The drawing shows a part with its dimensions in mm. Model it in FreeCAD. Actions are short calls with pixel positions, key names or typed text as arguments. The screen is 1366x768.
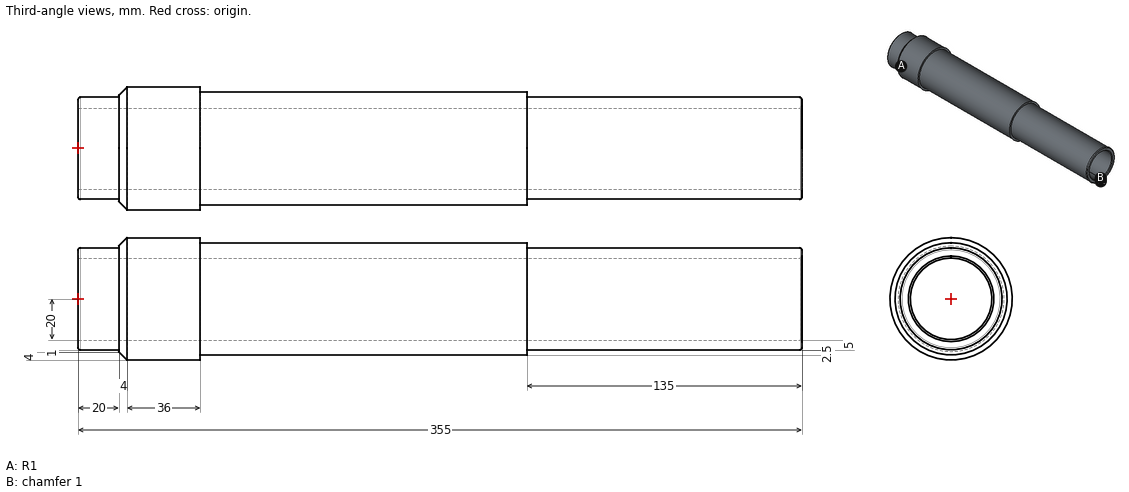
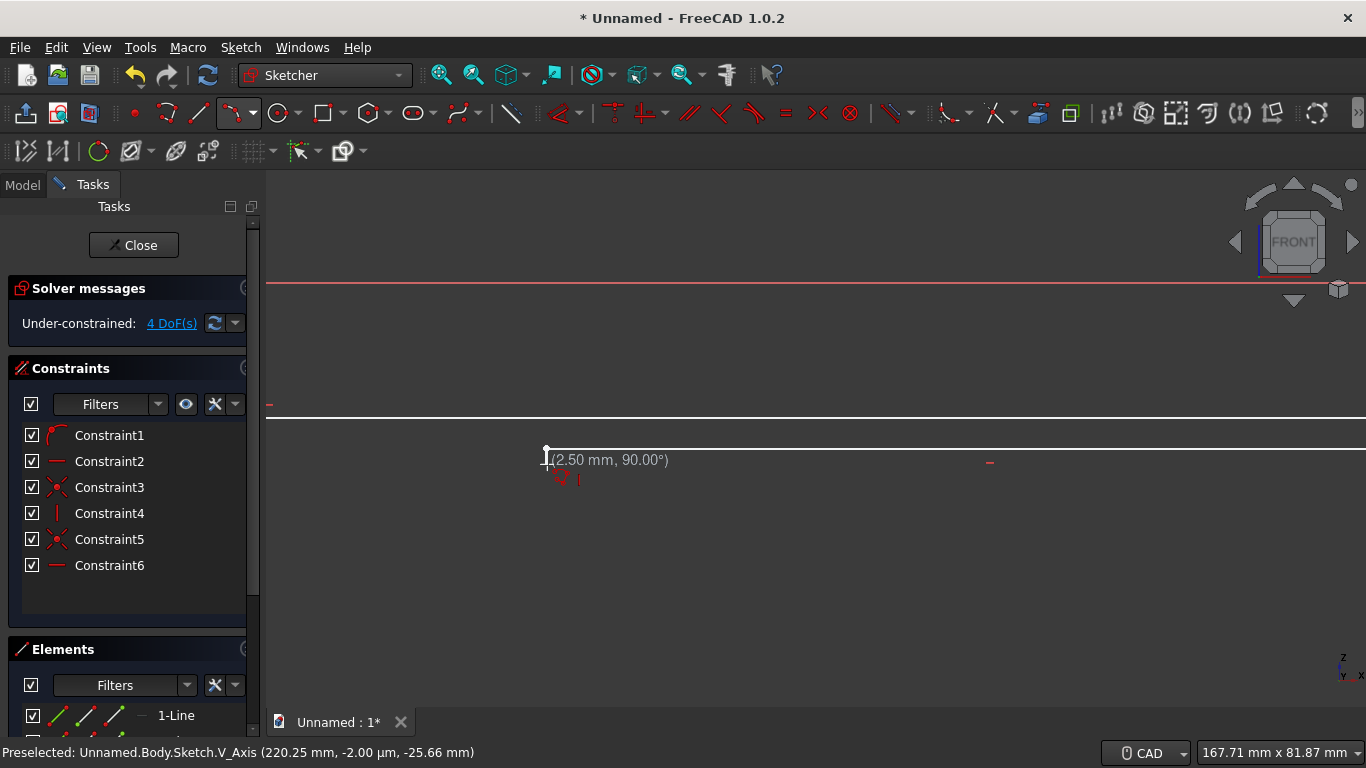
click(547, 463)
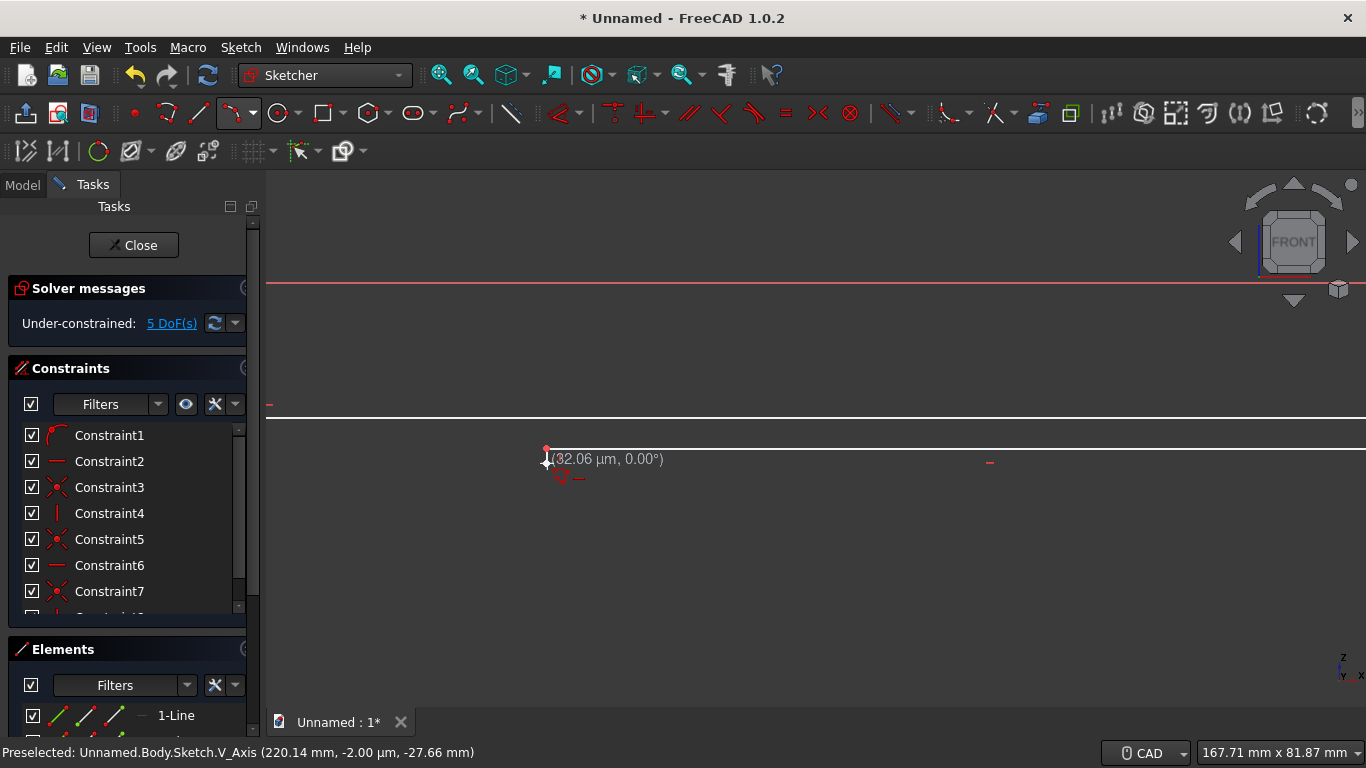
scroll(954, 463, down, 6)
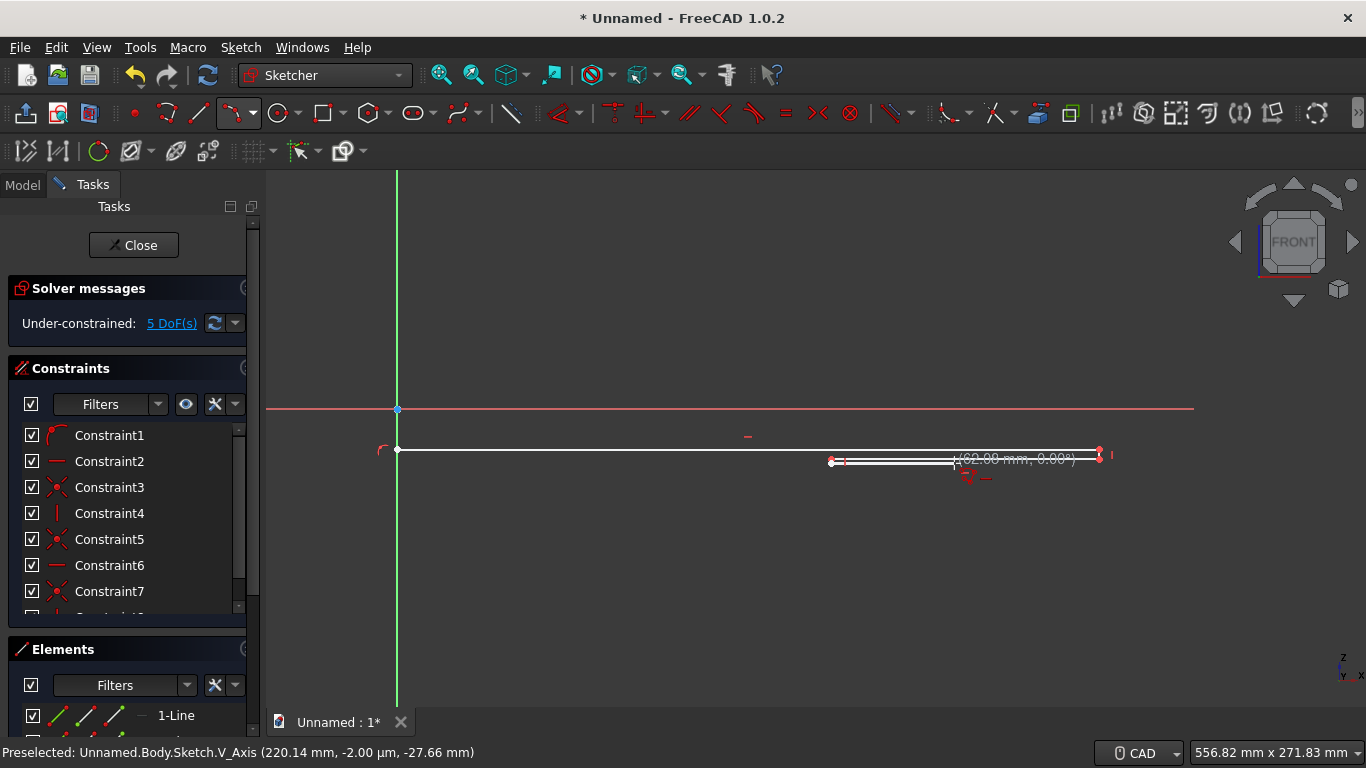
click(516, 463)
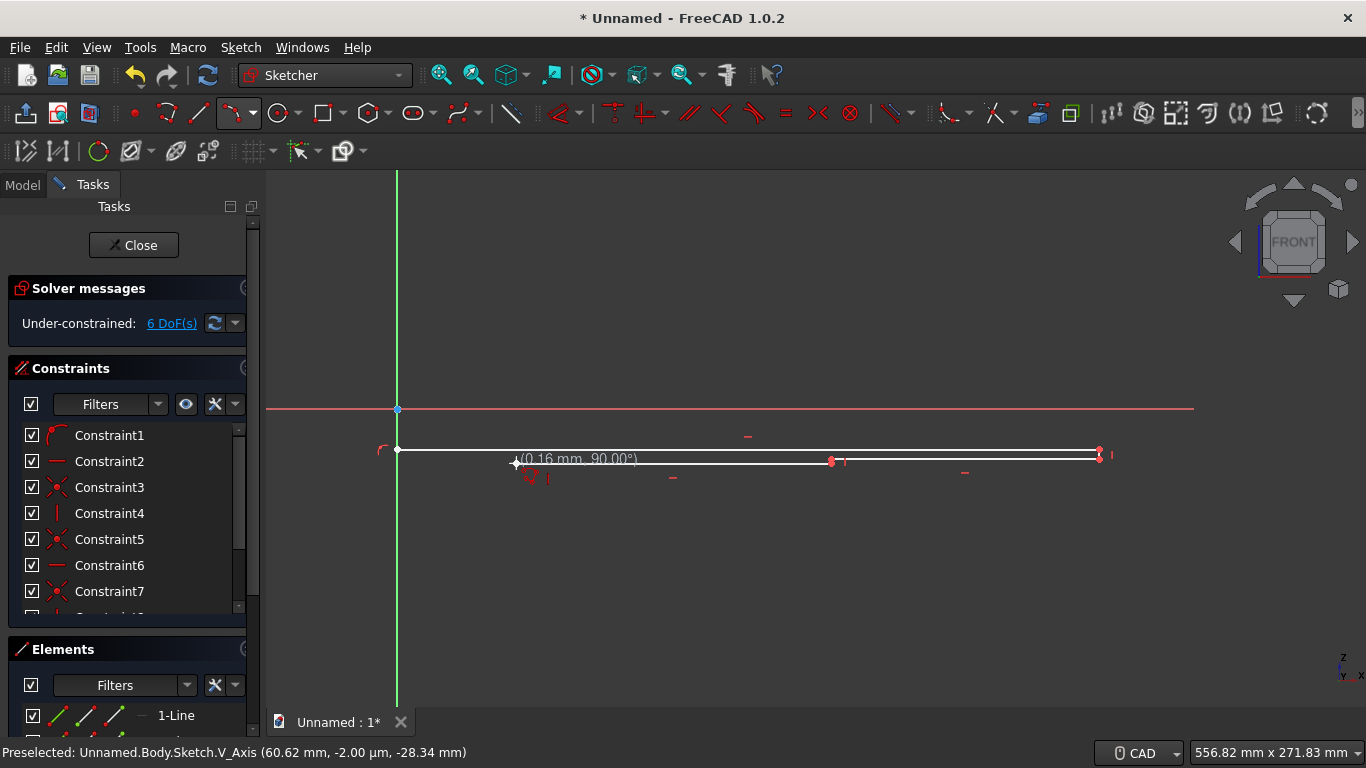
scroll(516, 468, up, 6)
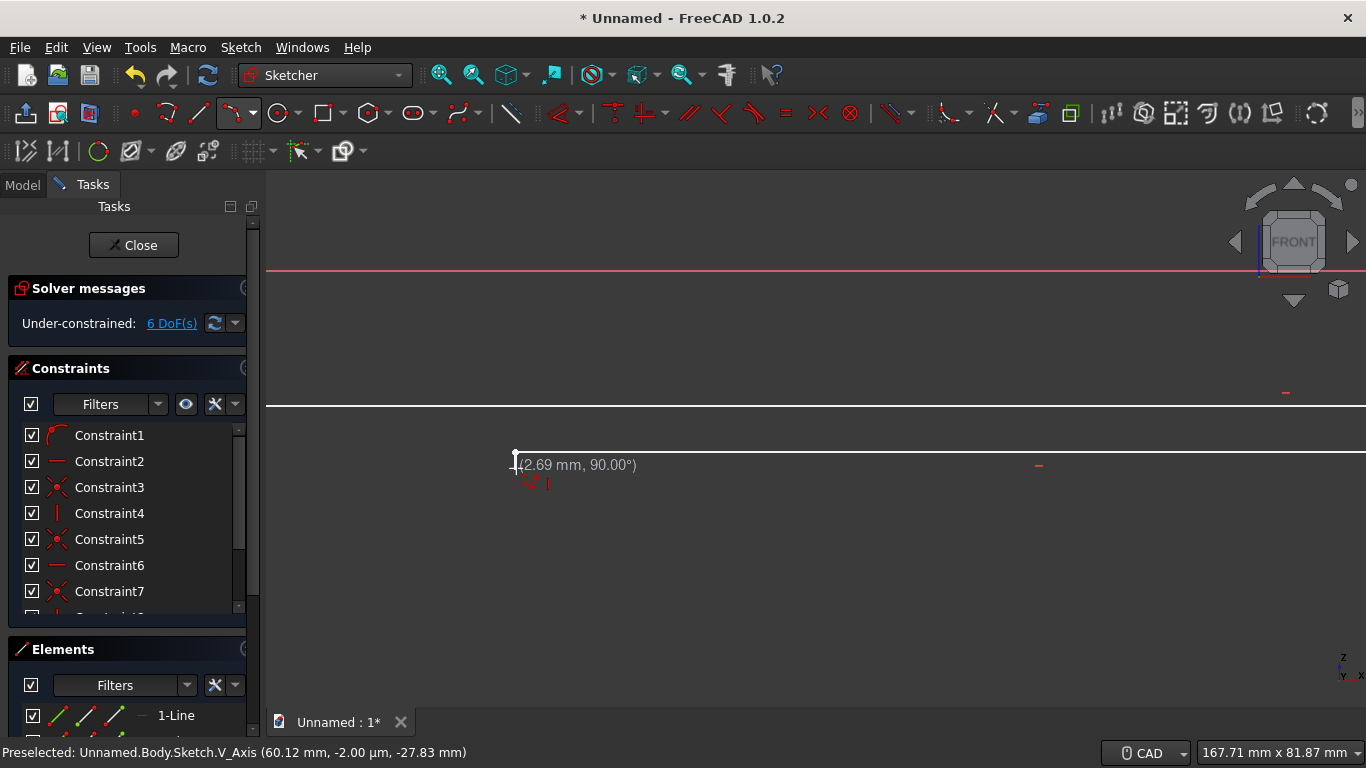
click(515, 468)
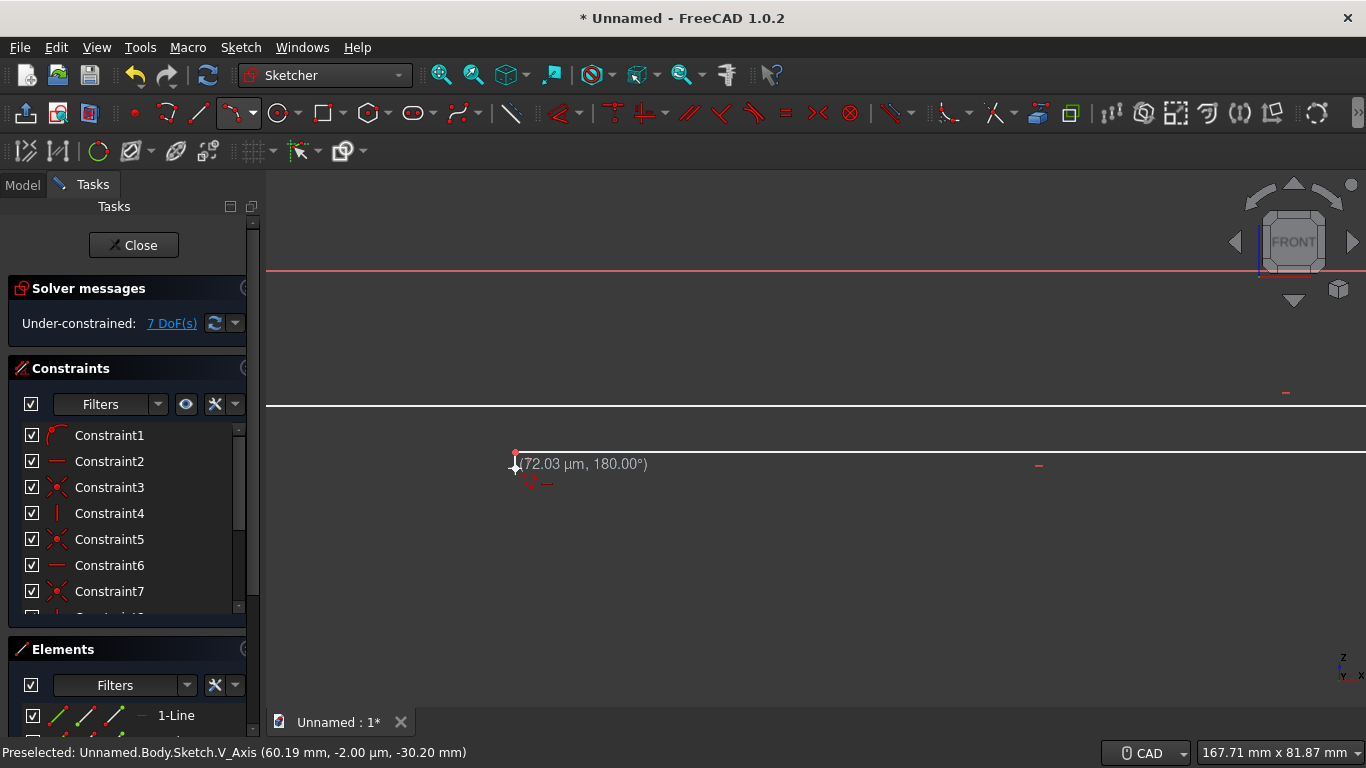
scroll(516, 468, down, 6)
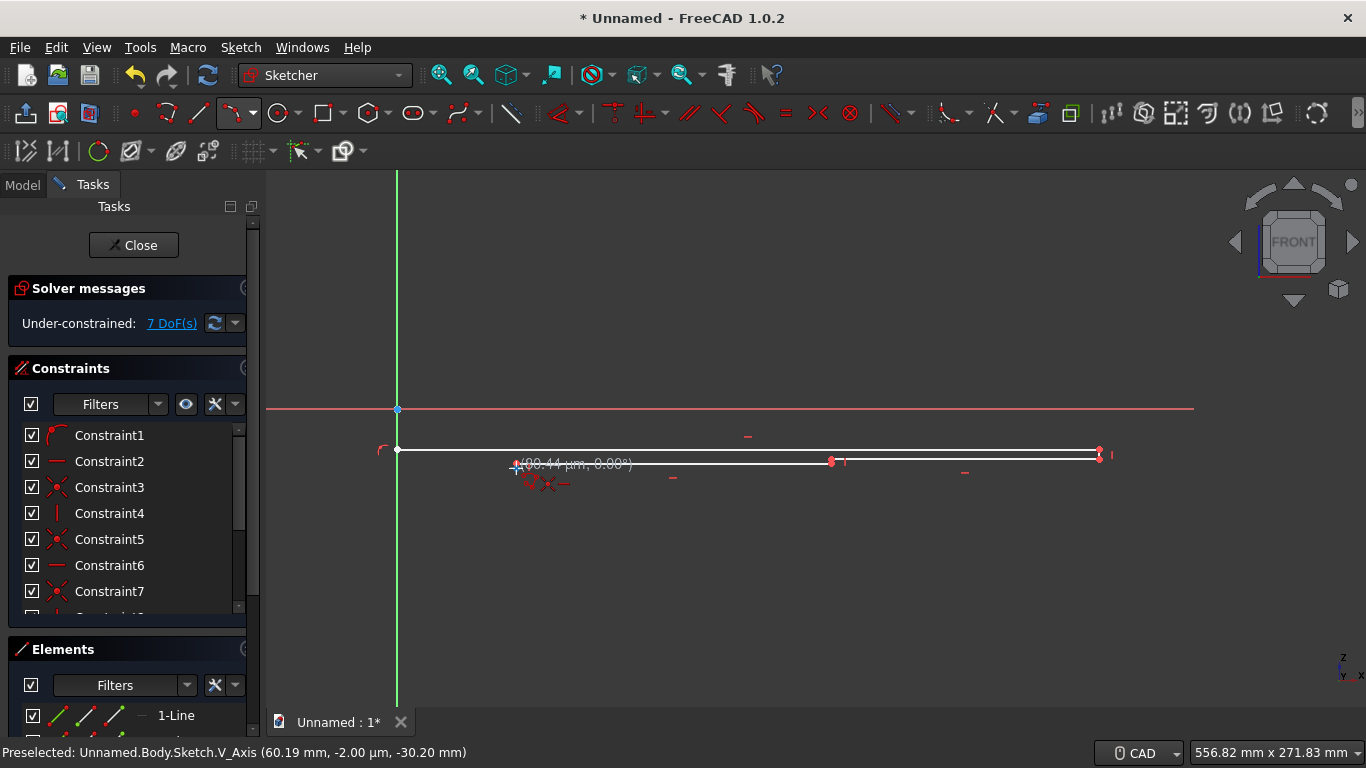
click(445, 468)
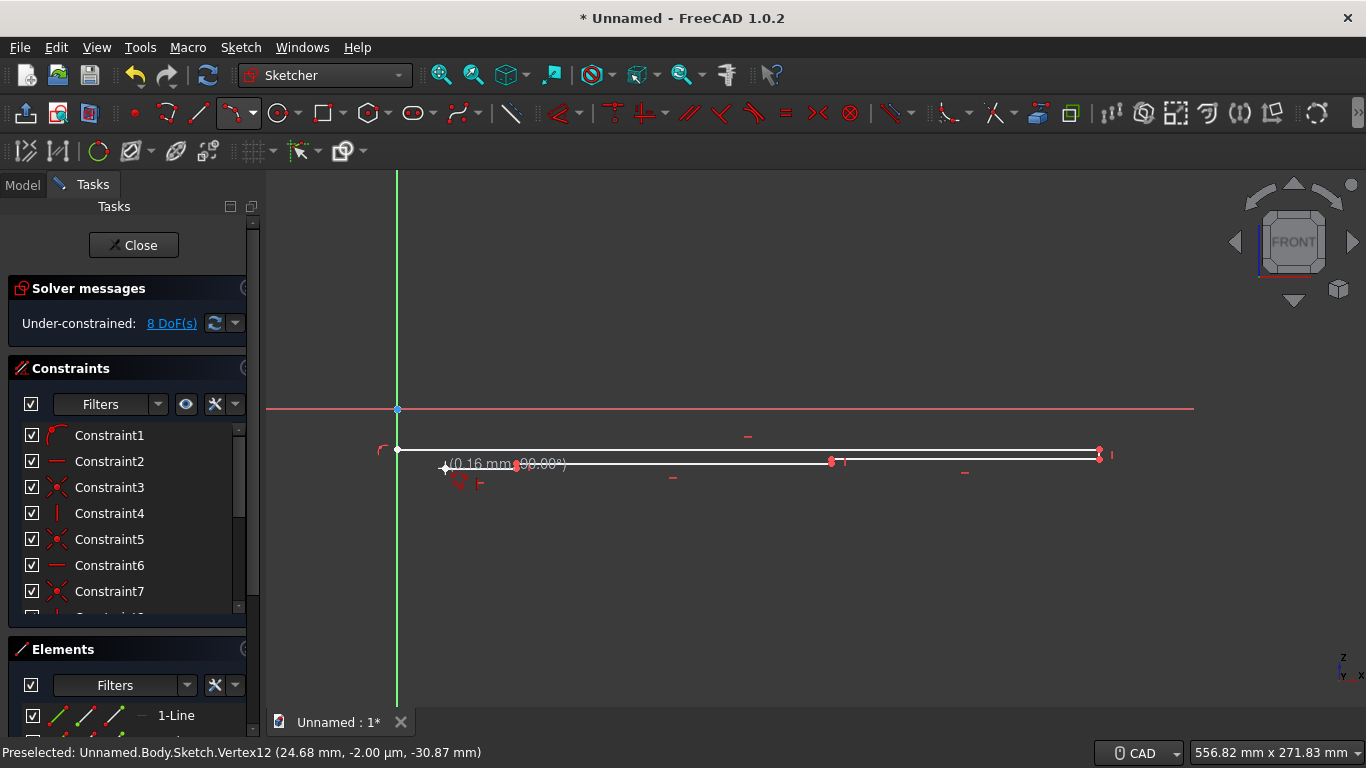
scroll(437, 460, up, 2)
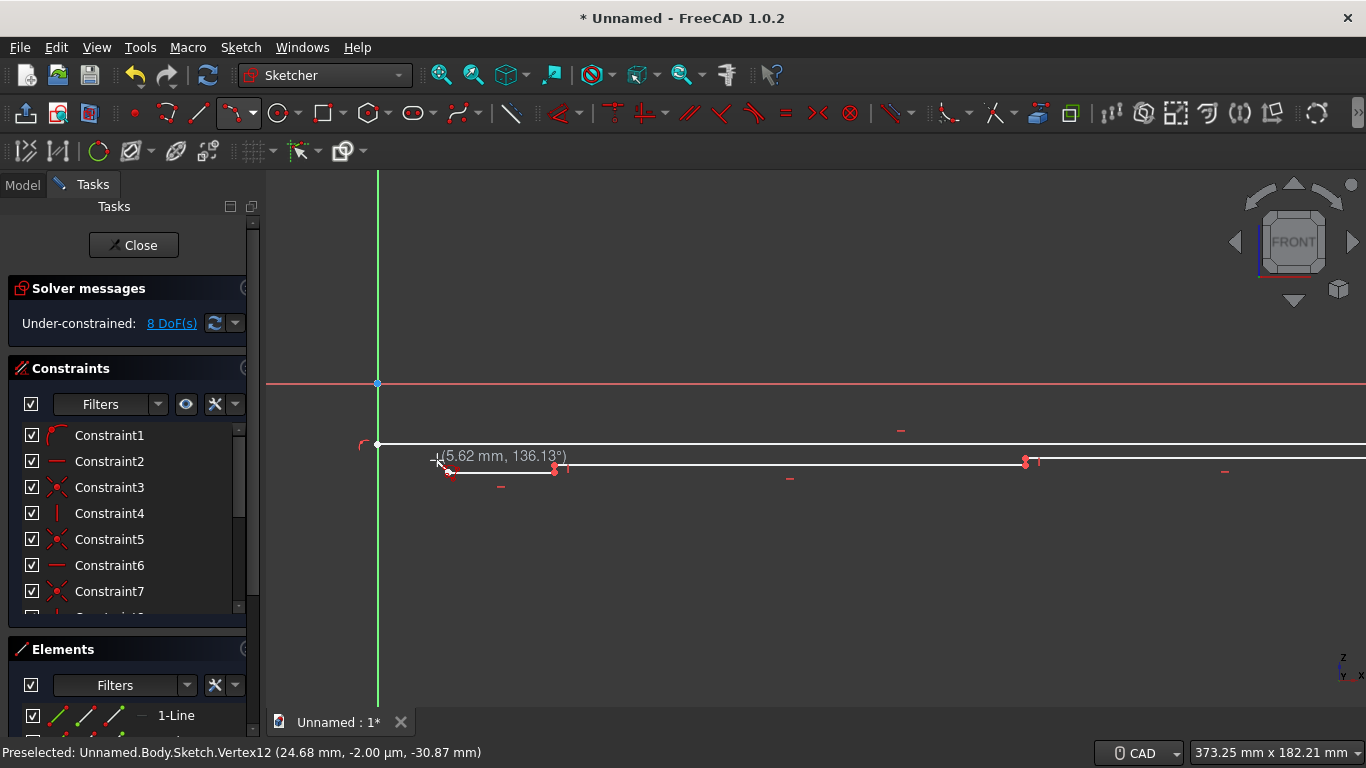
click(437, 460)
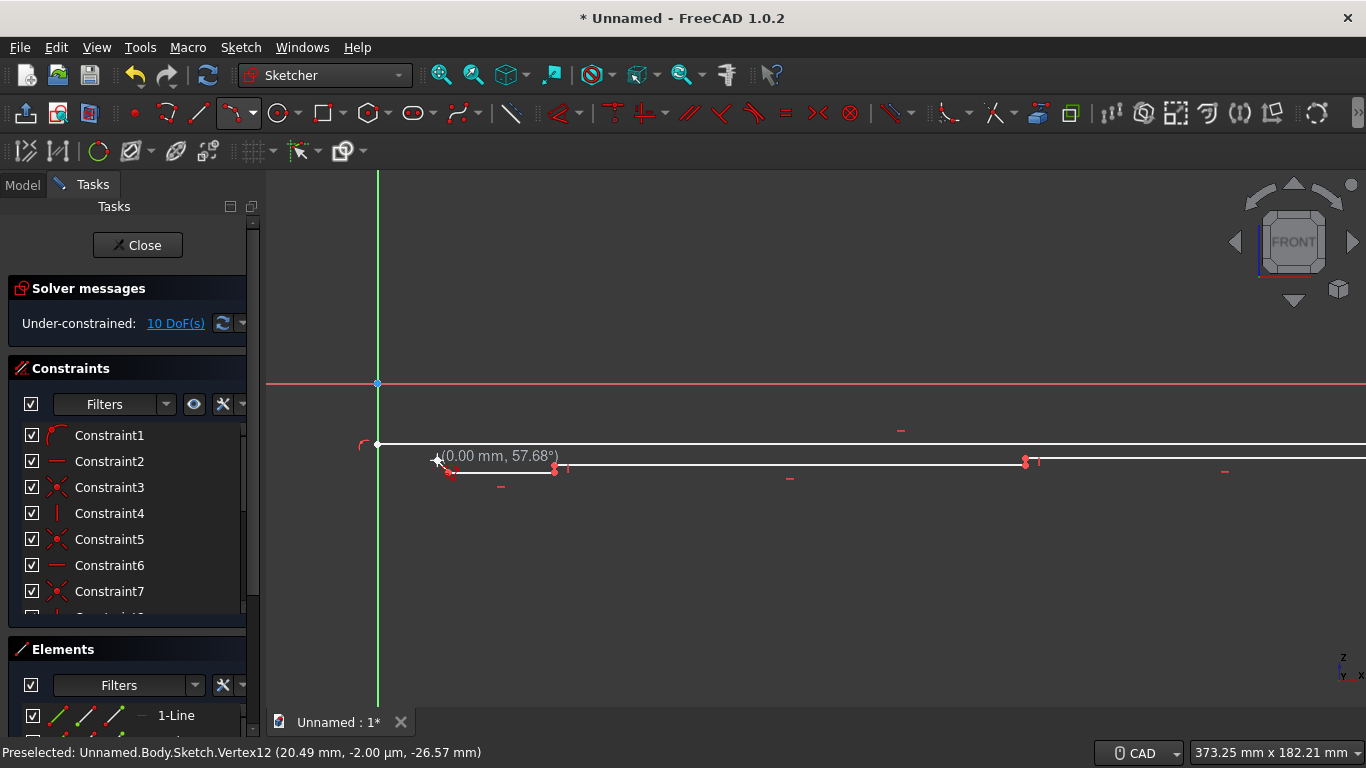
scroll(437, 457, up, 9)